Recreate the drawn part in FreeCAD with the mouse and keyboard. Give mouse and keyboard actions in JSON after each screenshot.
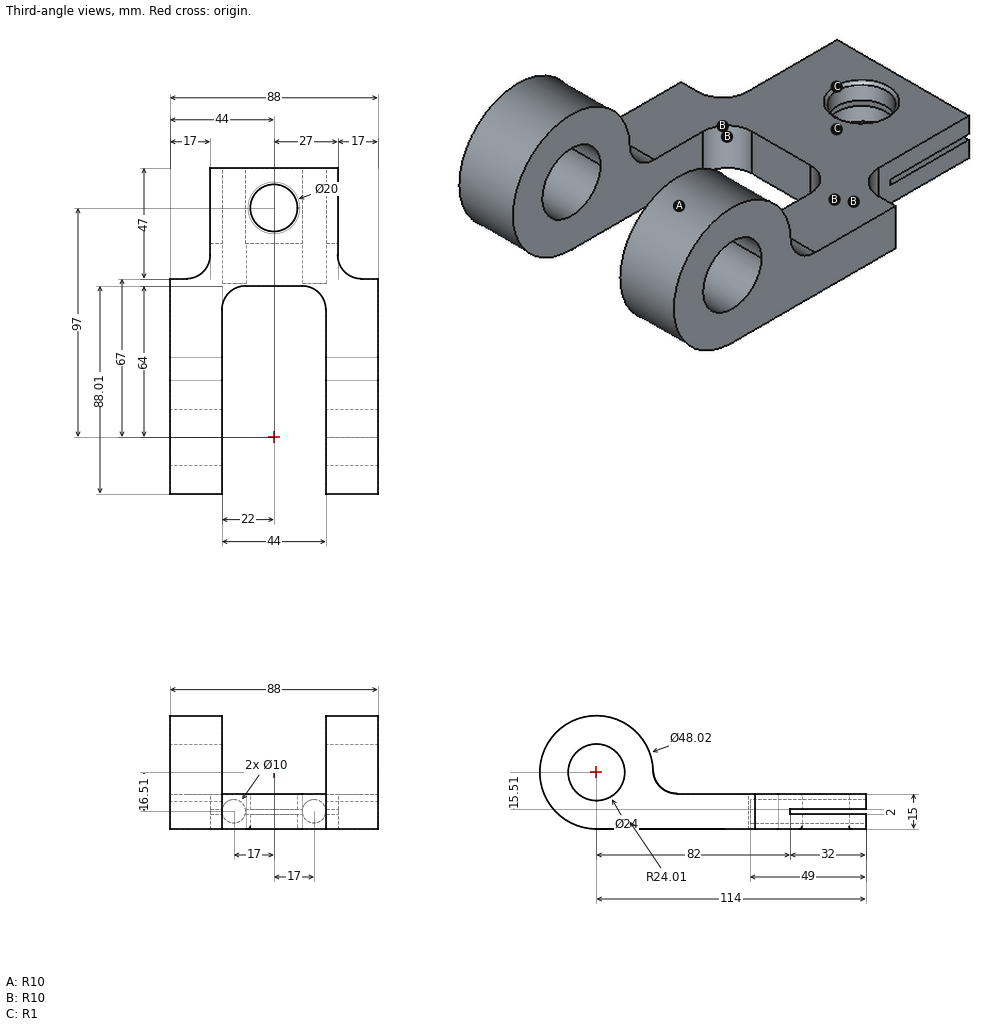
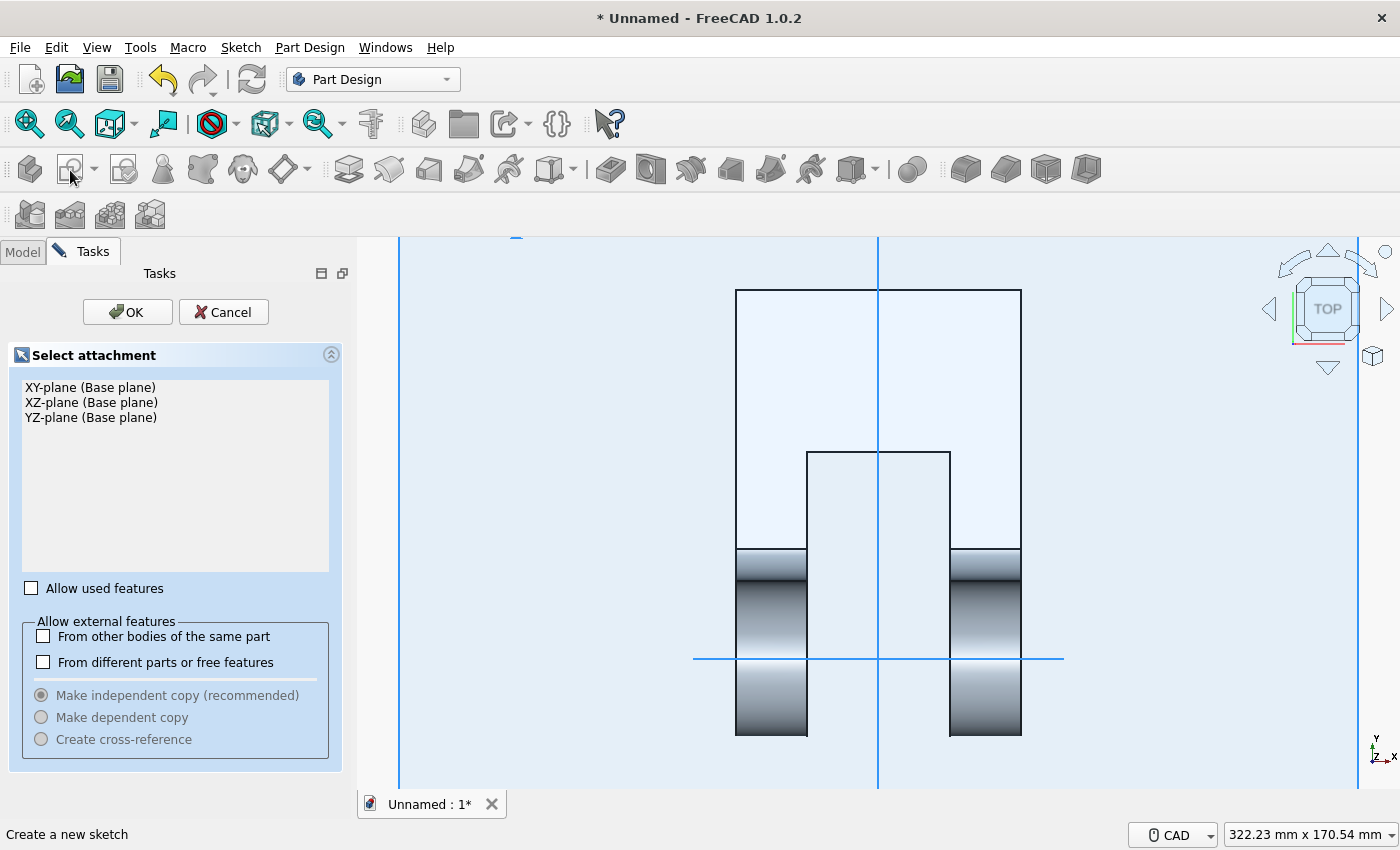
{"action": "left_click", "coordinate": [82, 388]}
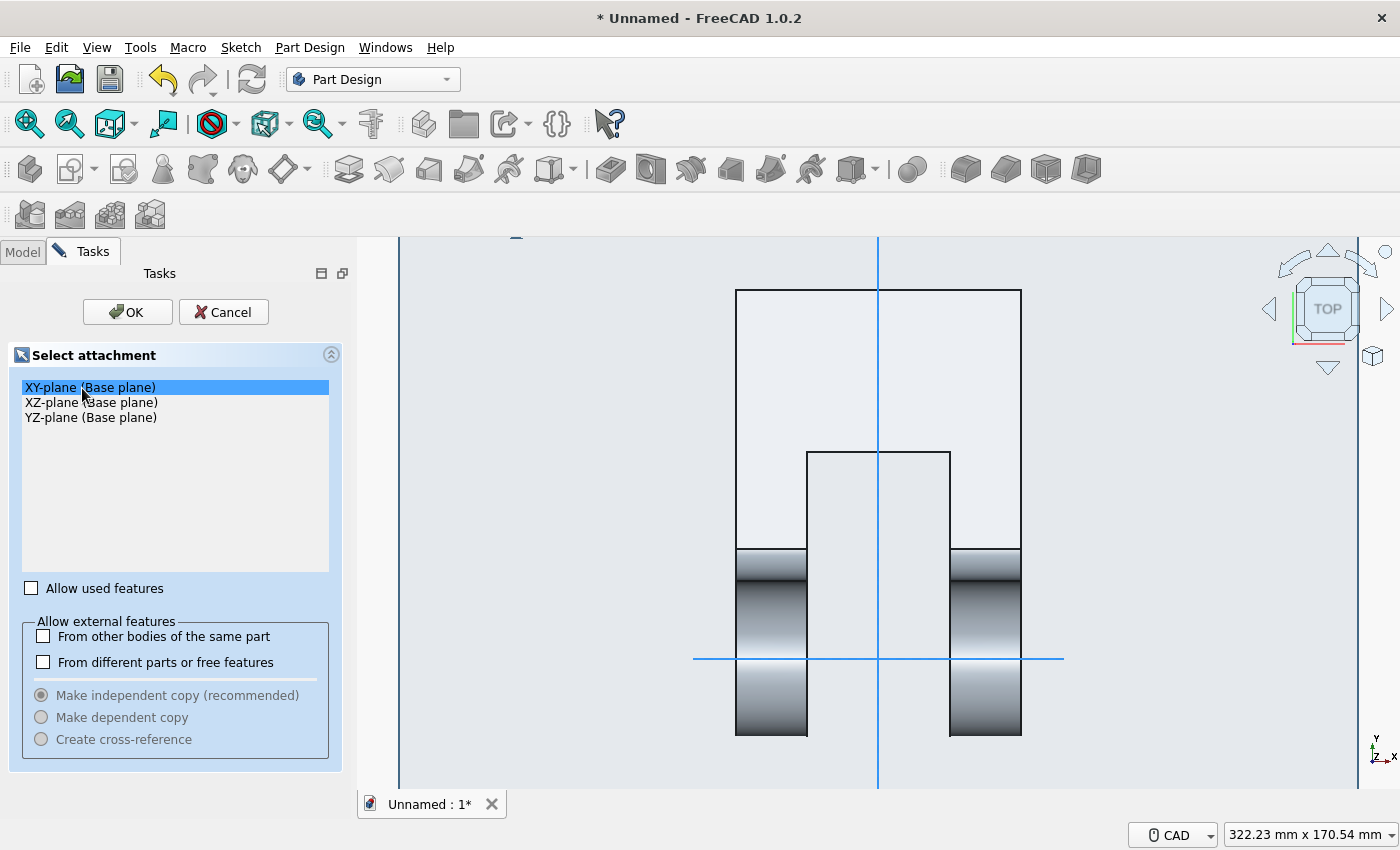
{"action": "left_click", "coordinate": [128, 312]}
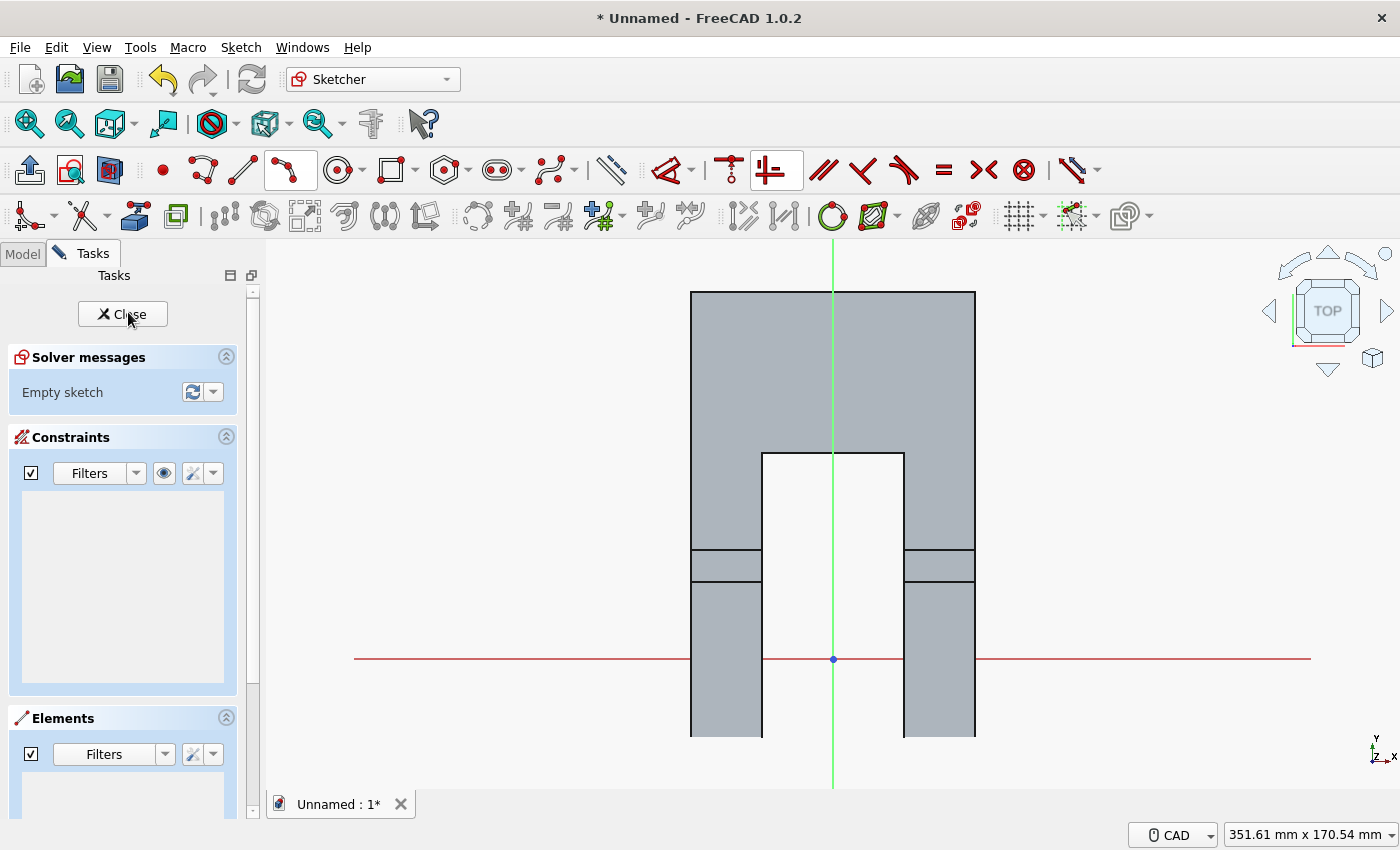
{"action": "left_click", "coordinate": [110, 170]}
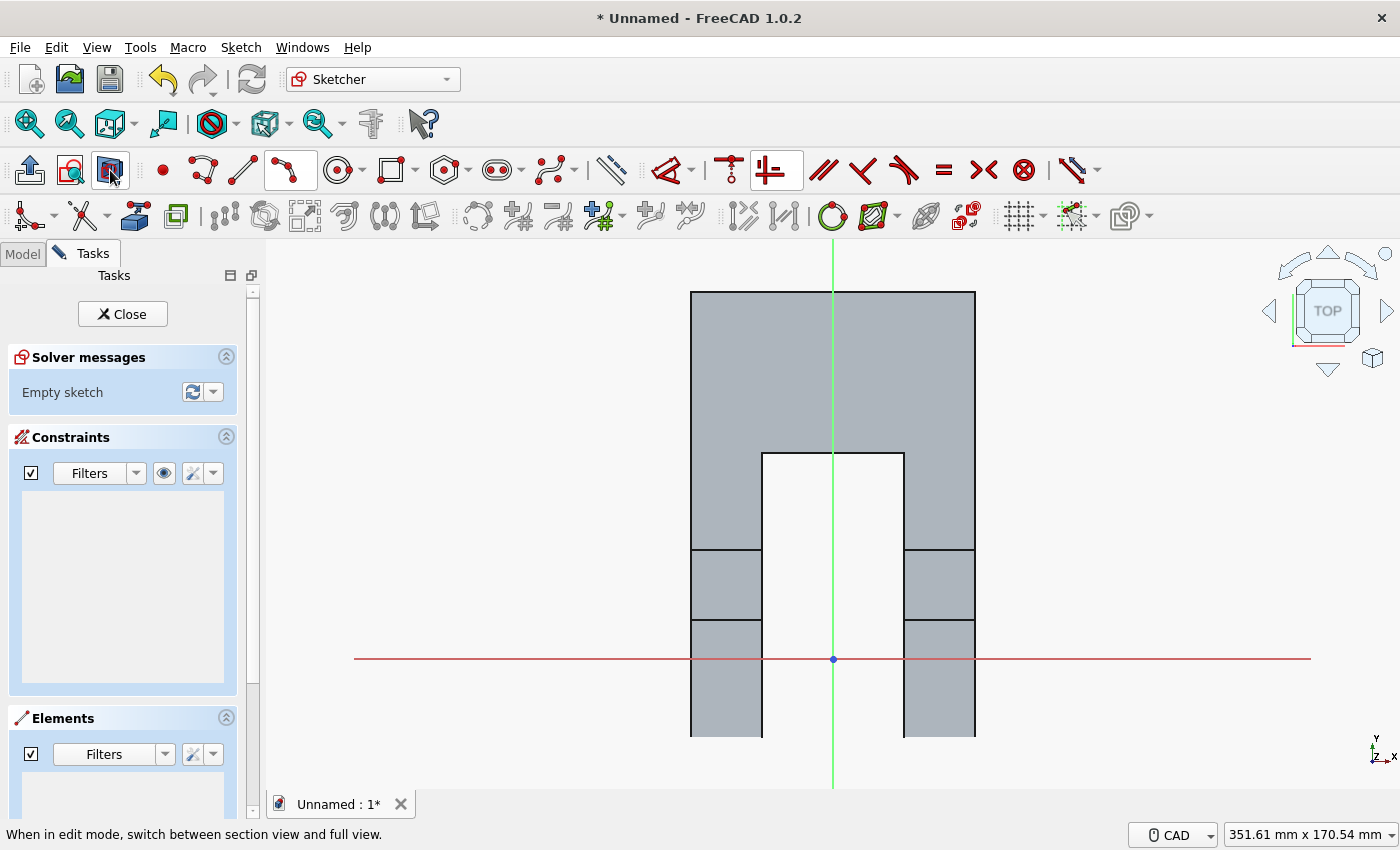
{"action": "scroll", "coordinate": [455, 689], "scroll_direction": "down", "scroll_amount": 1}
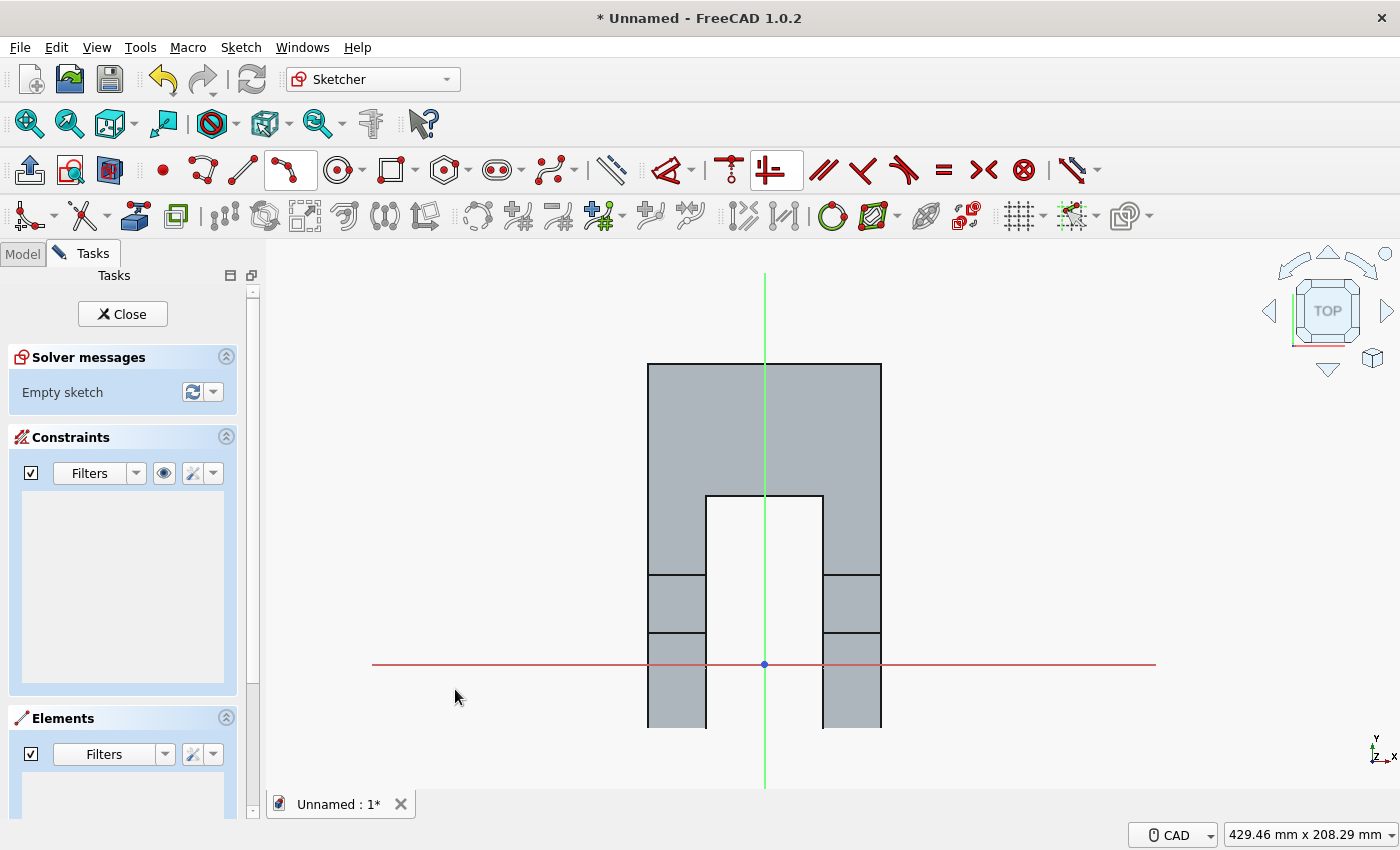
{"action": "left_click", "coordinate": [392, 170]}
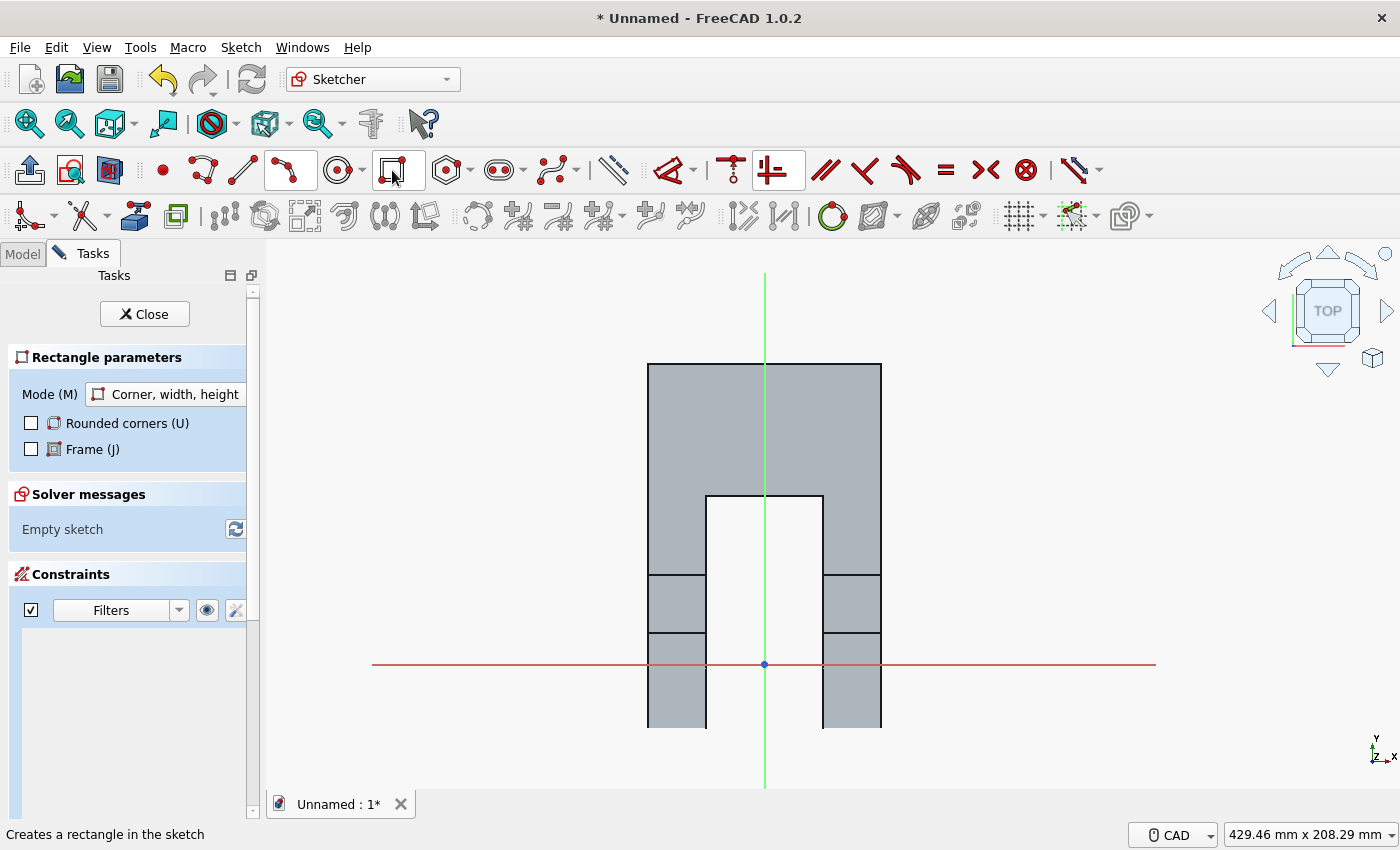
{"action": "left_click", "coordinate": [648, 364]}
{"action": "left_click", "coordinate": [693, 488]}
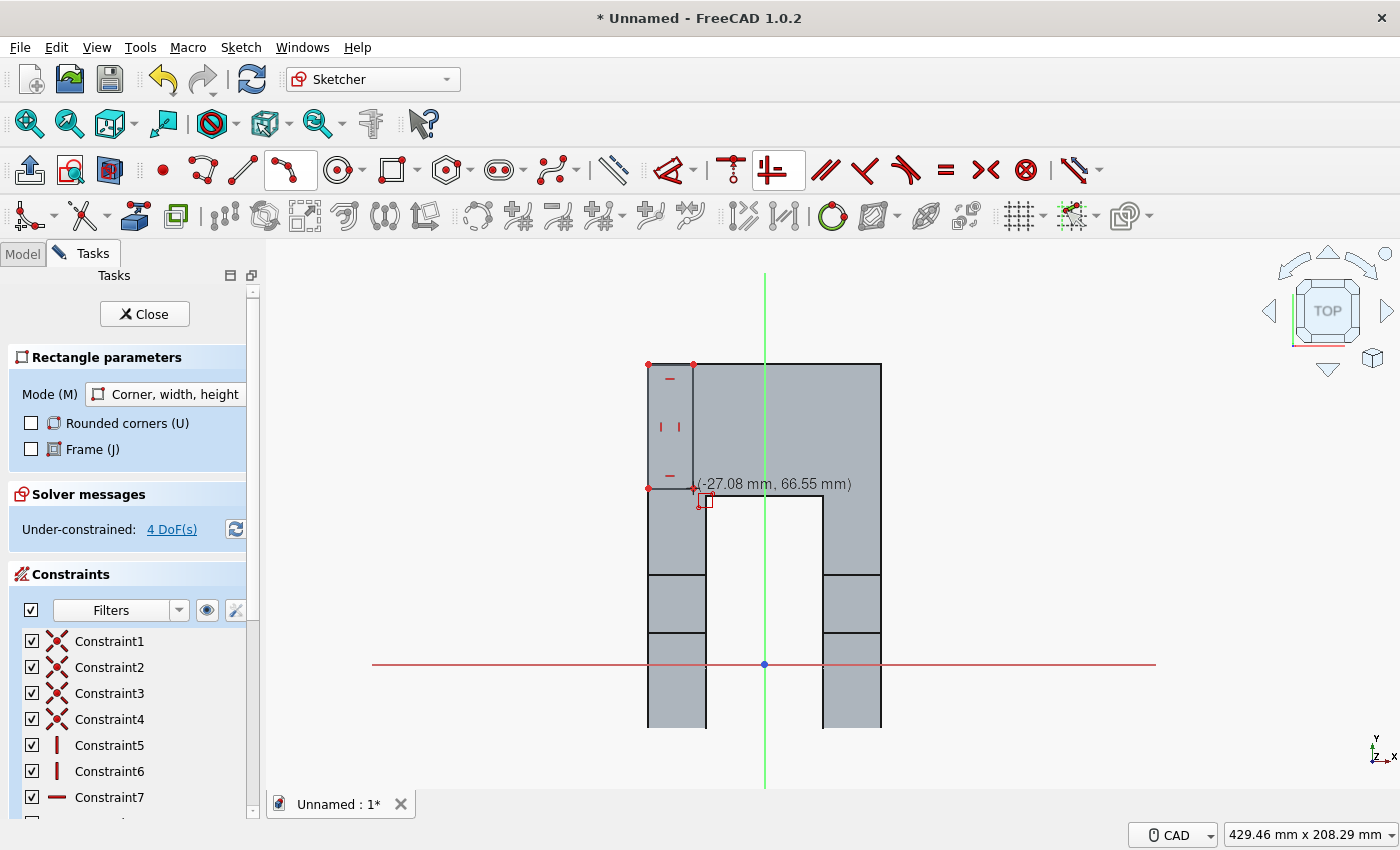
{"action": "left_click", "coordinate": [836, 364]}
{"action": "left_click", "coordinate": [881, 488]}
{"action": "key", "text": "Escape"}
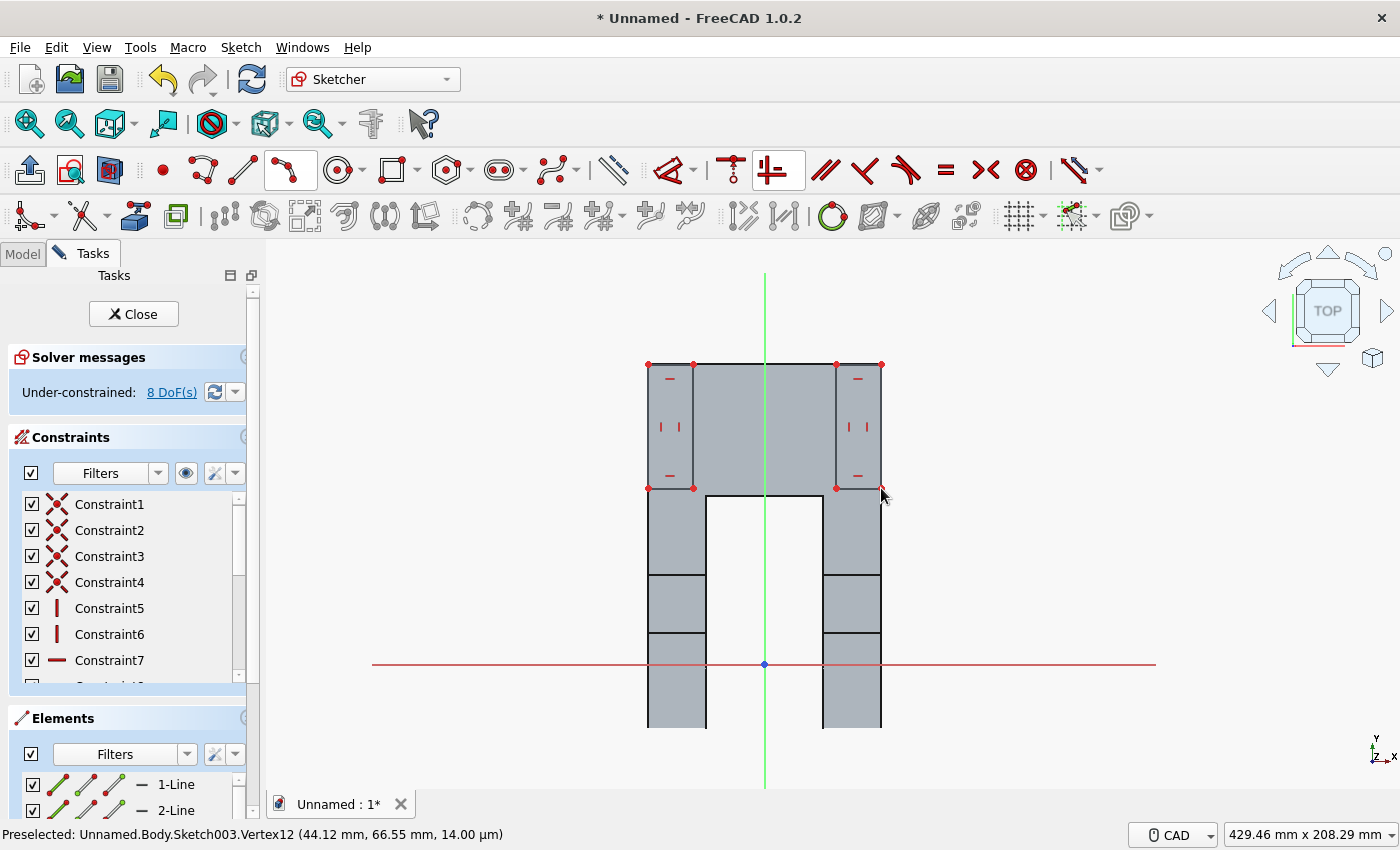
{"action": "left_click", "coordinate": [668, 170]}